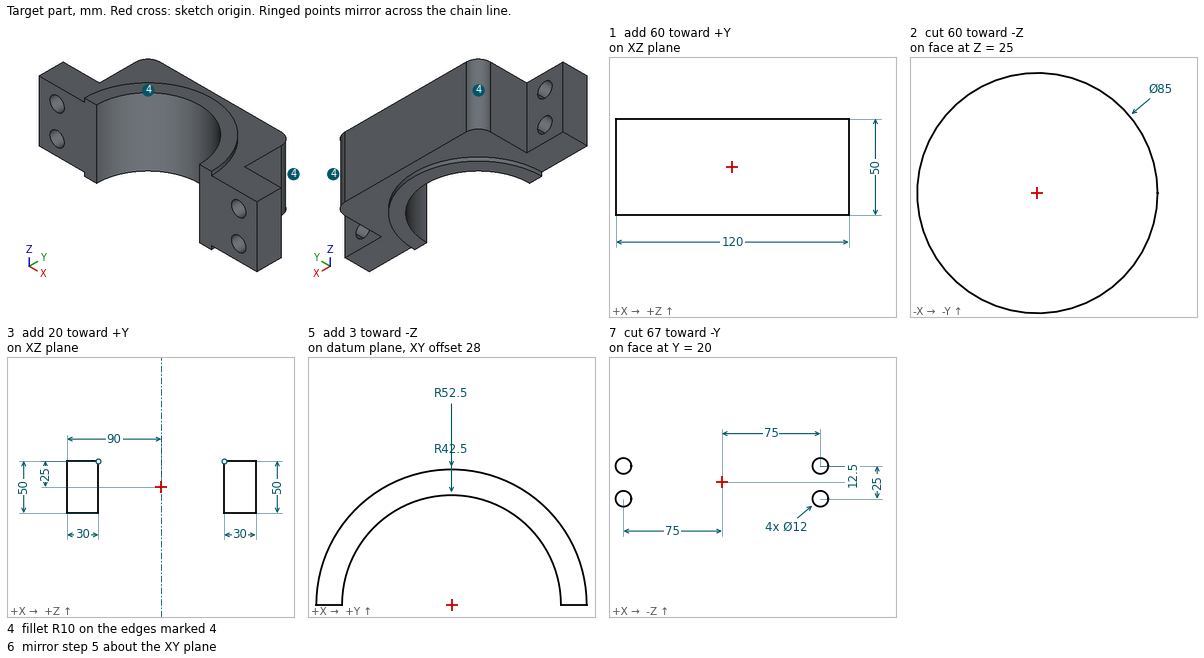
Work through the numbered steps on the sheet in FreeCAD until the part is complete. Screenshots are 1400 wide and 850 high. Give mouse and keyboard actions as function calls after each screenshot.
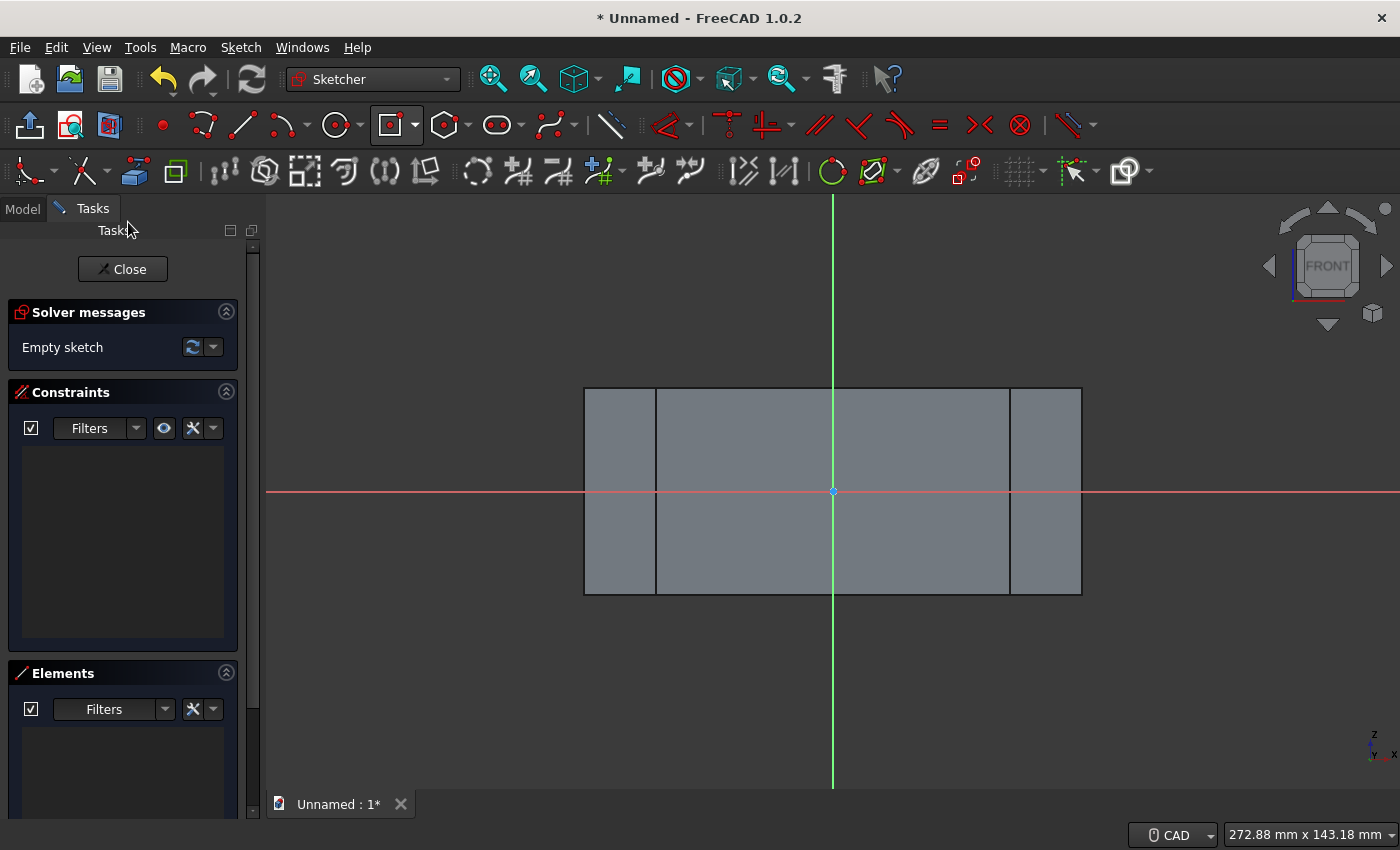
click(418, 126)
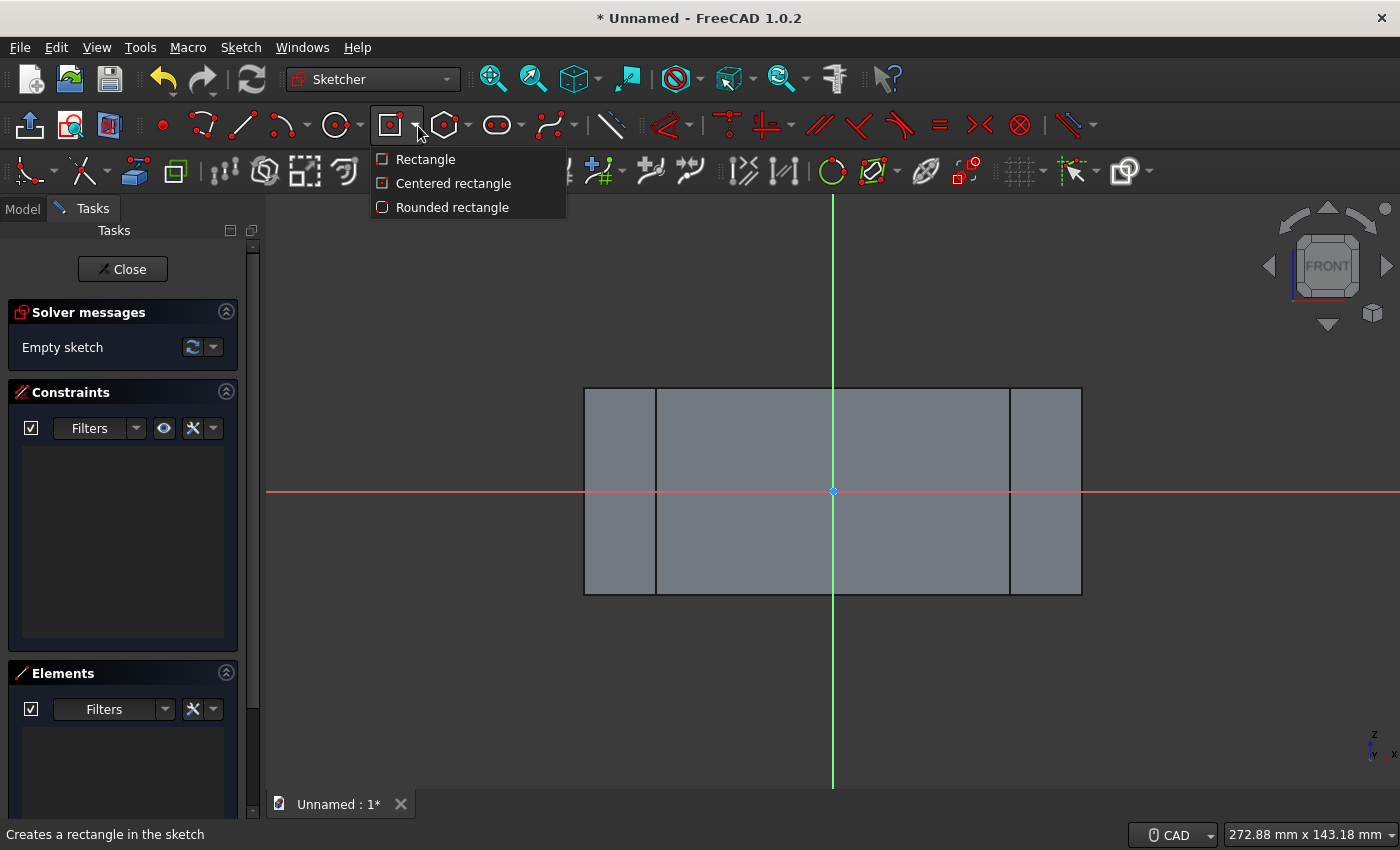
click(468, 159)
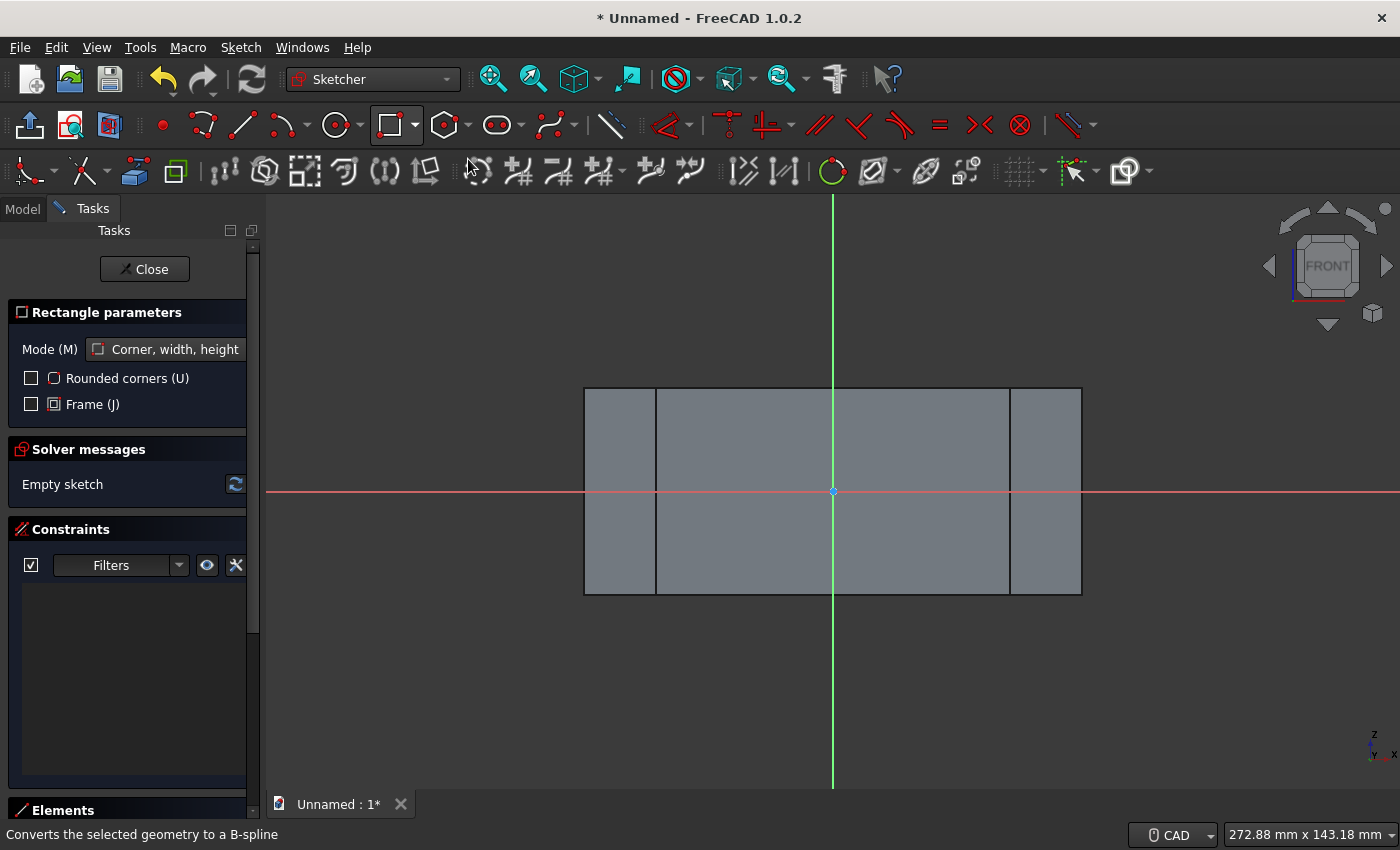
click(459, 388)
move(584, 595)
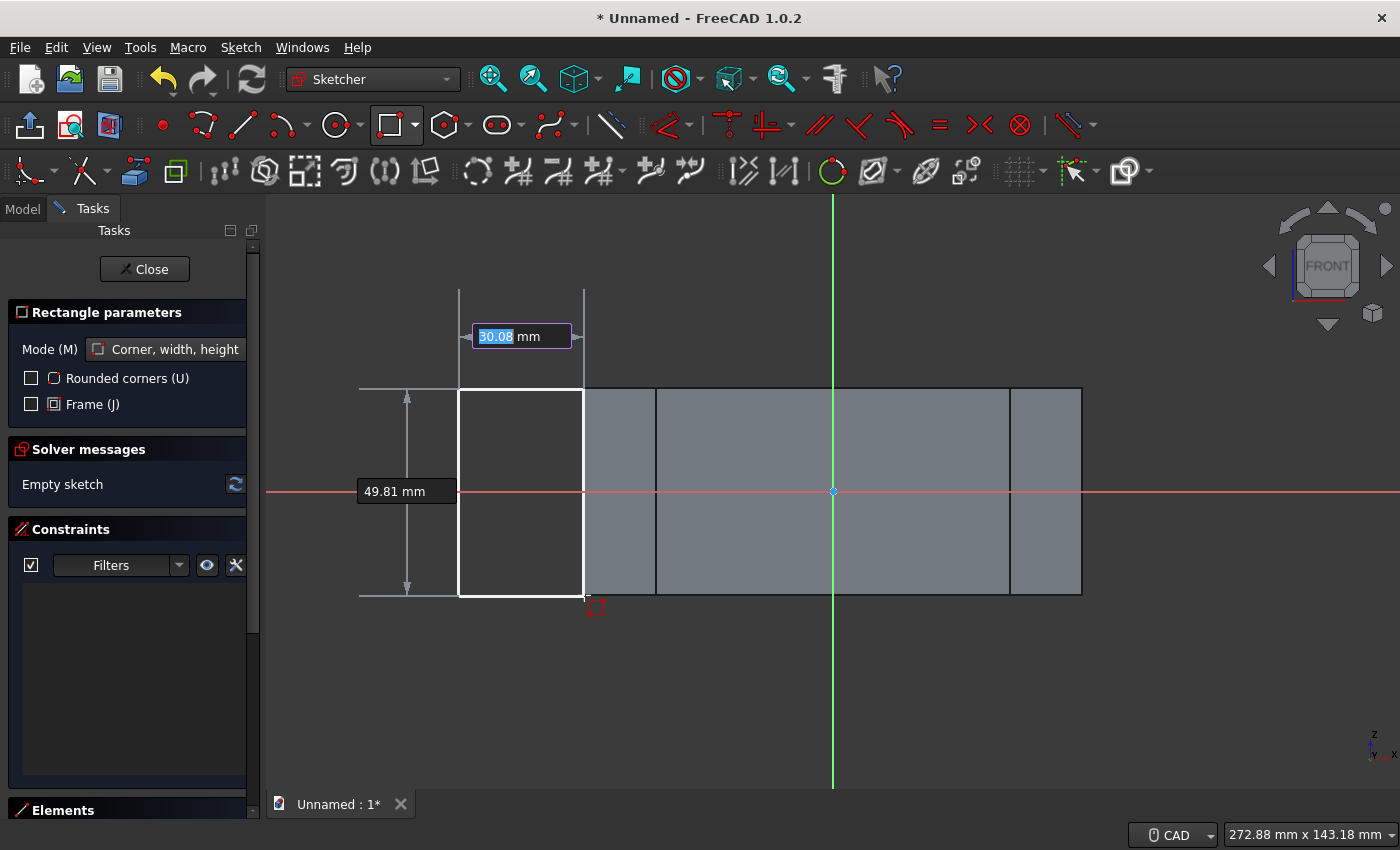
text(30)
key(Tab)
text(50)
key(Return)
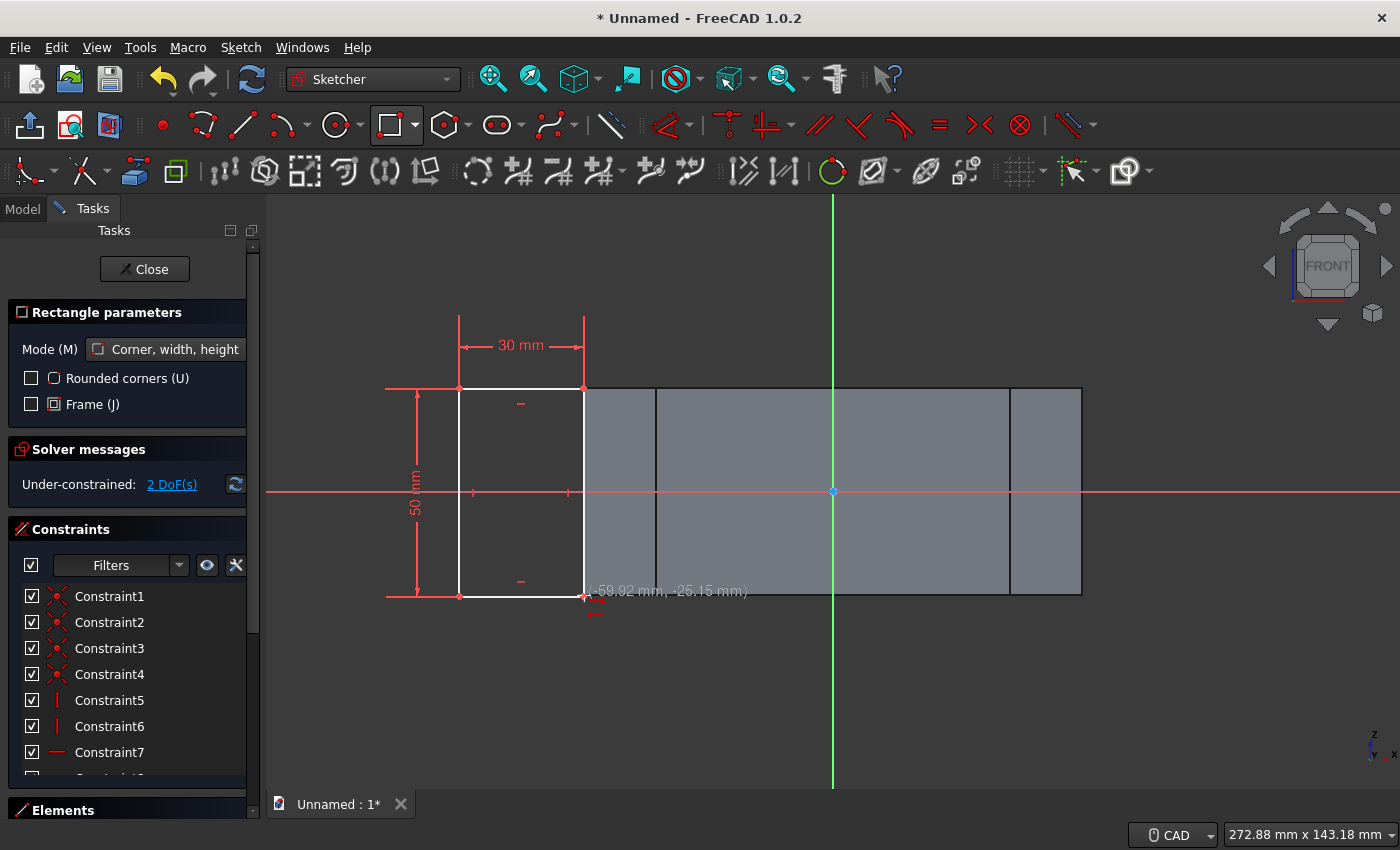
click(1082, 388)
move(1207, 595)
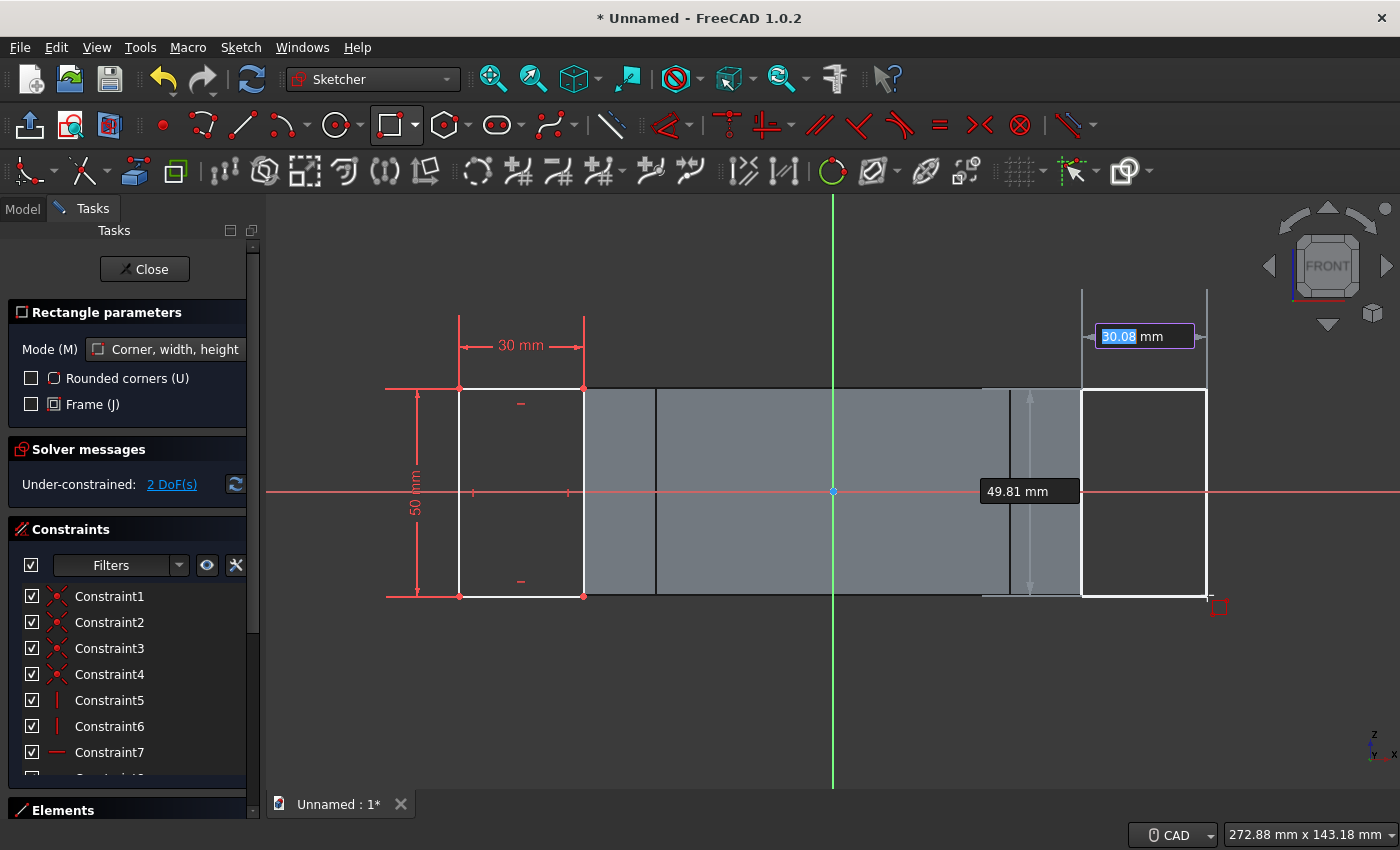
text(30)
key(Tab)
text(50)
key(Return)
key(Escape)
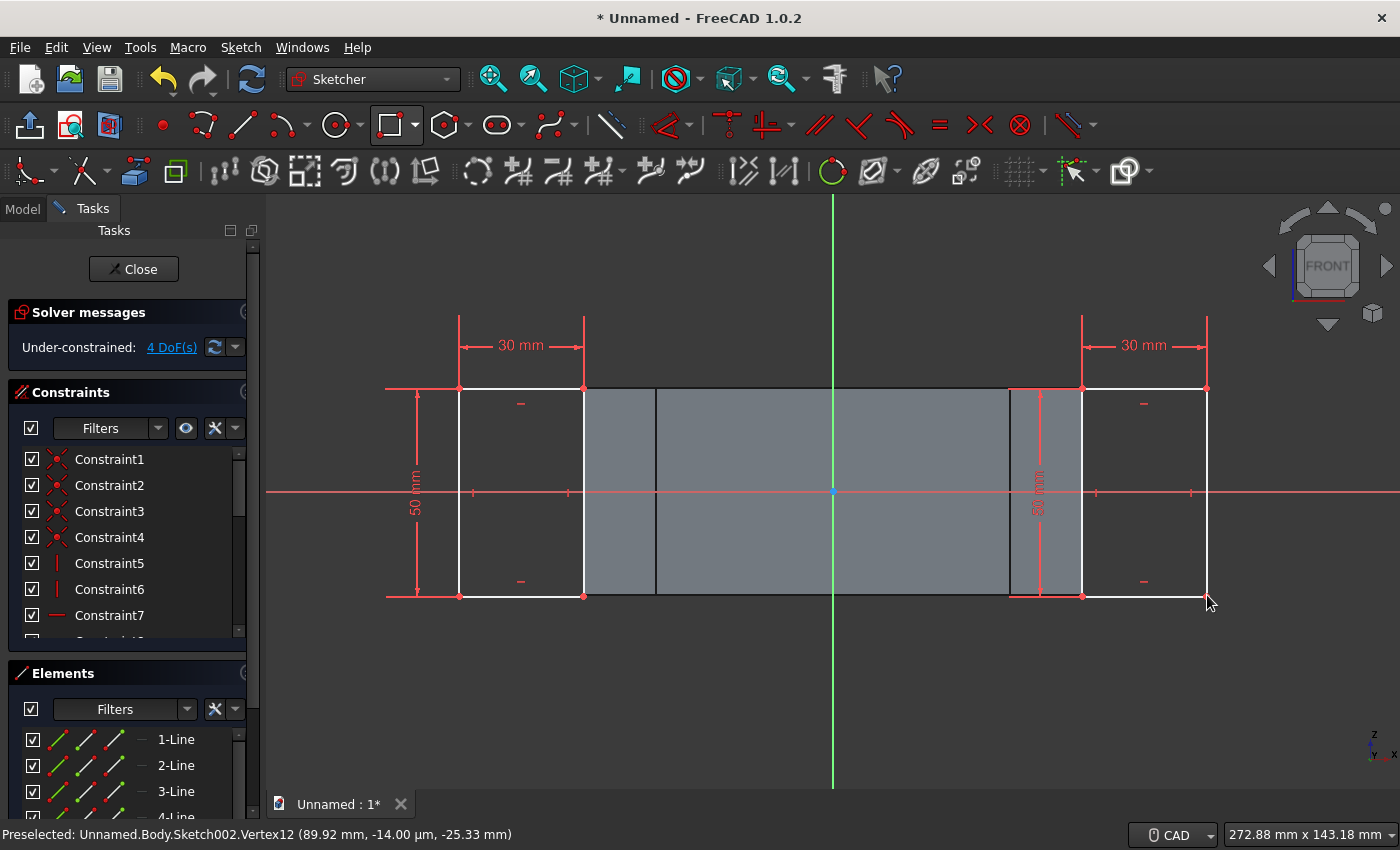
click(584, 389)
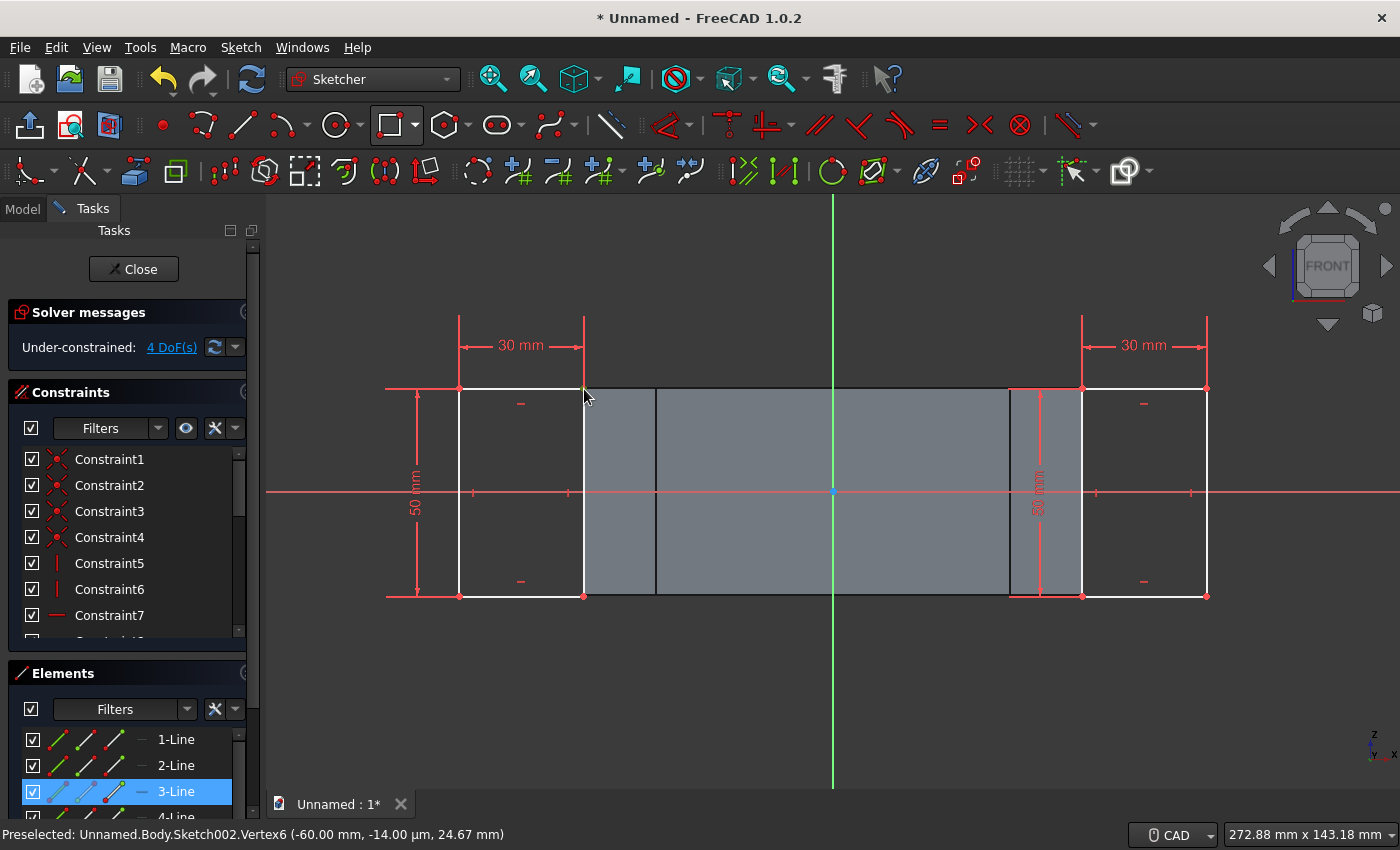
click(1082, 389)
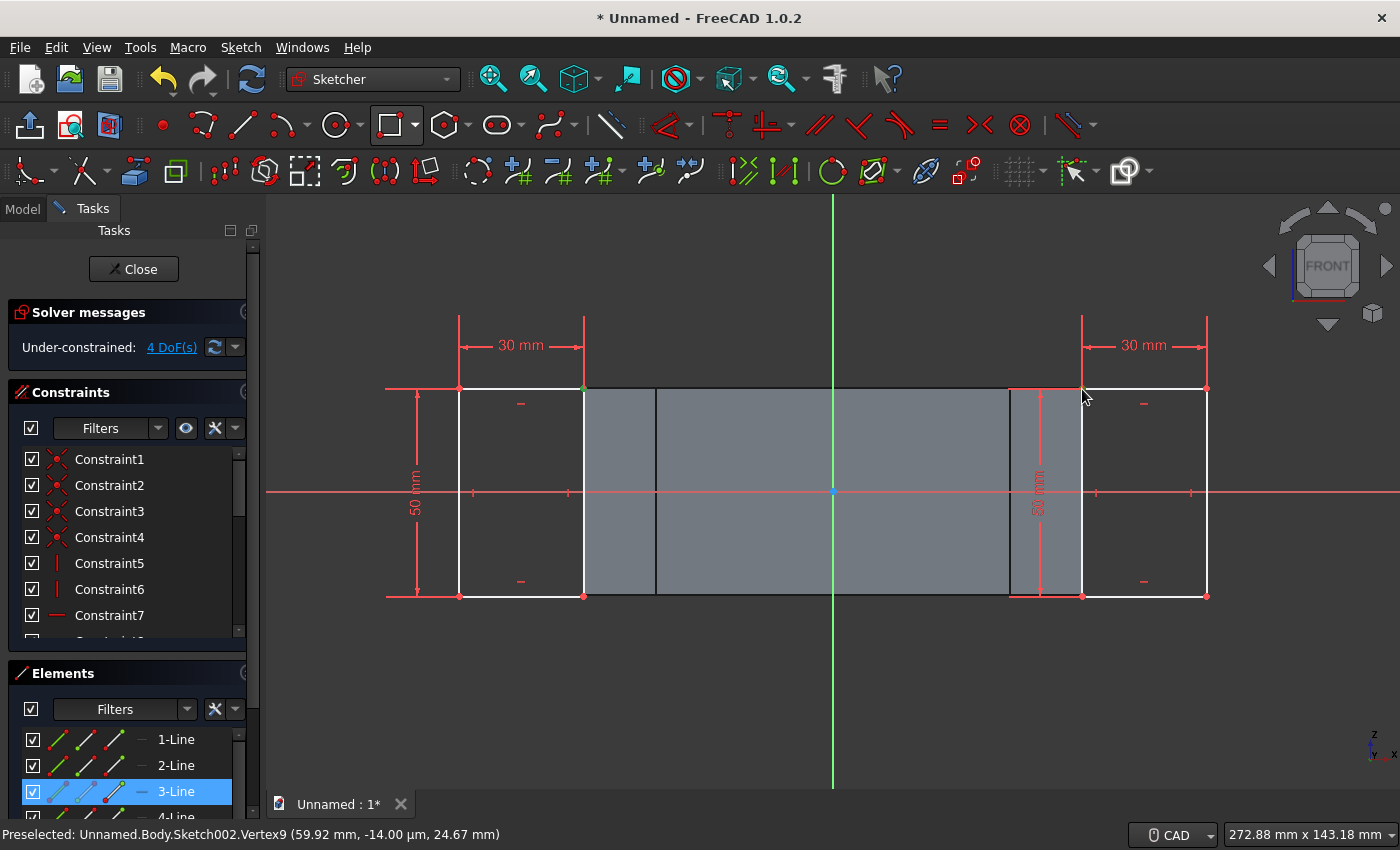
click(833, 722)